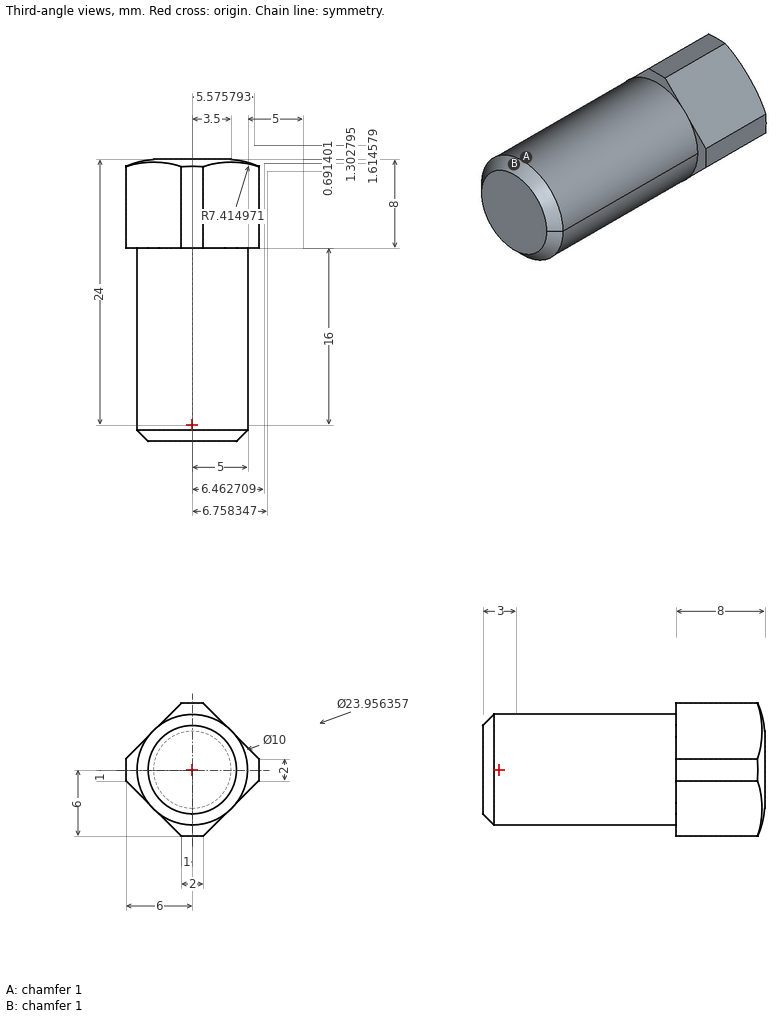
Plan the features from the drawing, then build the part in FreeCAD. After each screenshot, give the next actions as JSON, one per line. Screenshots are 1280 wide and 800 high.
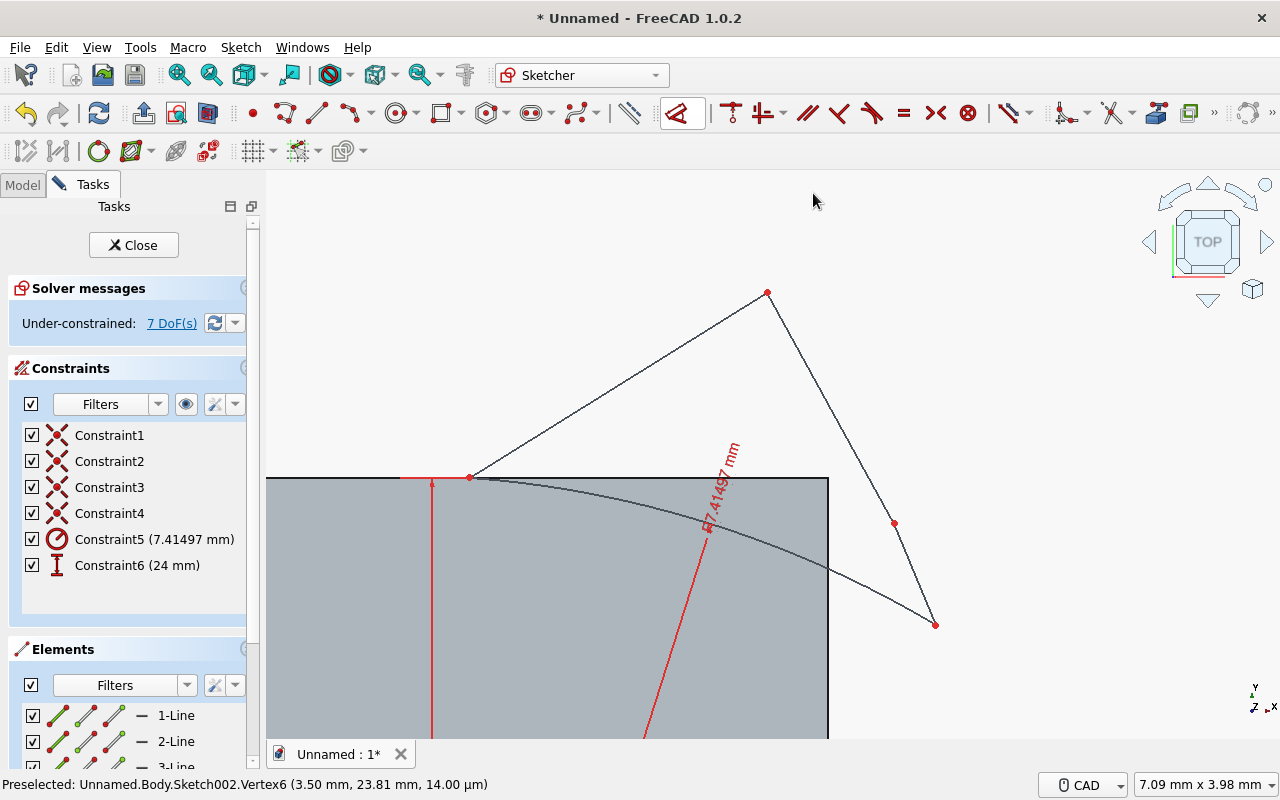
{"action": "left_click", "coordinate": [470, 478]}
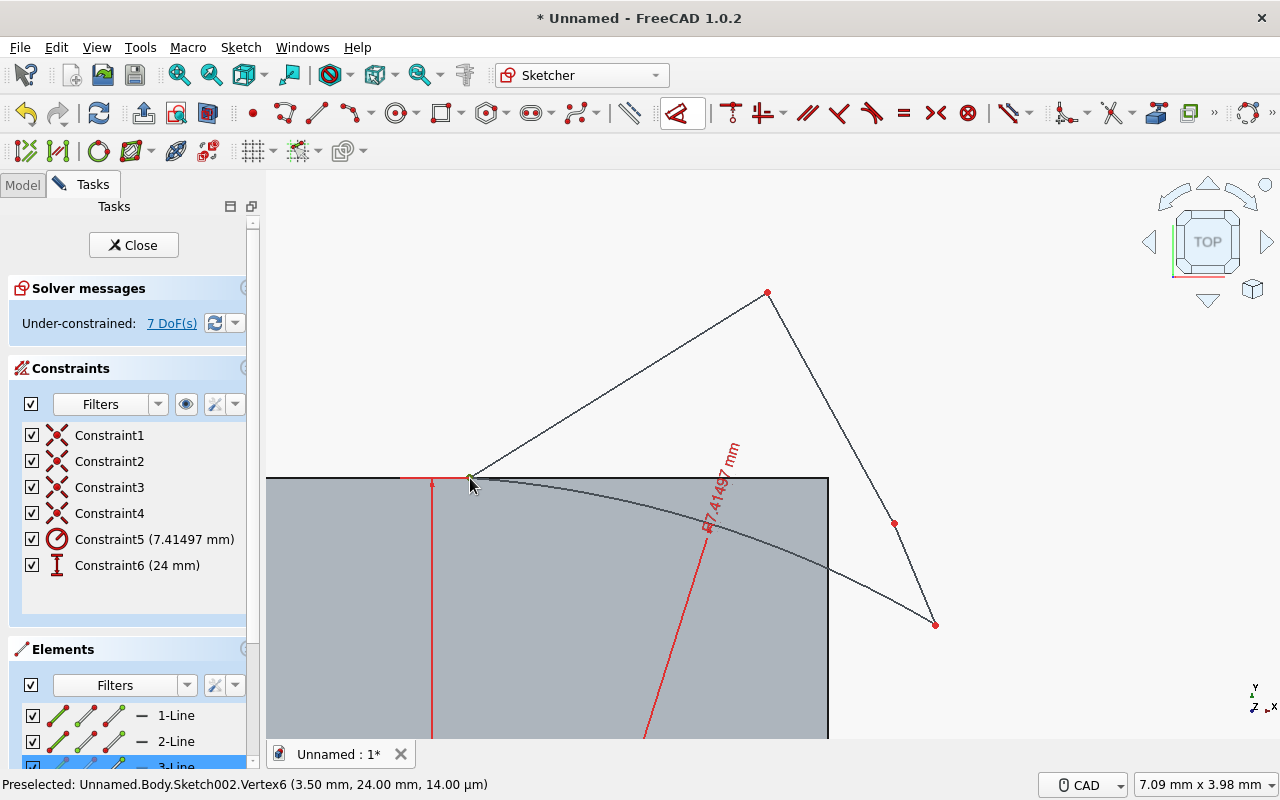
{"action": "left_click", "coordinate": [700, 114]}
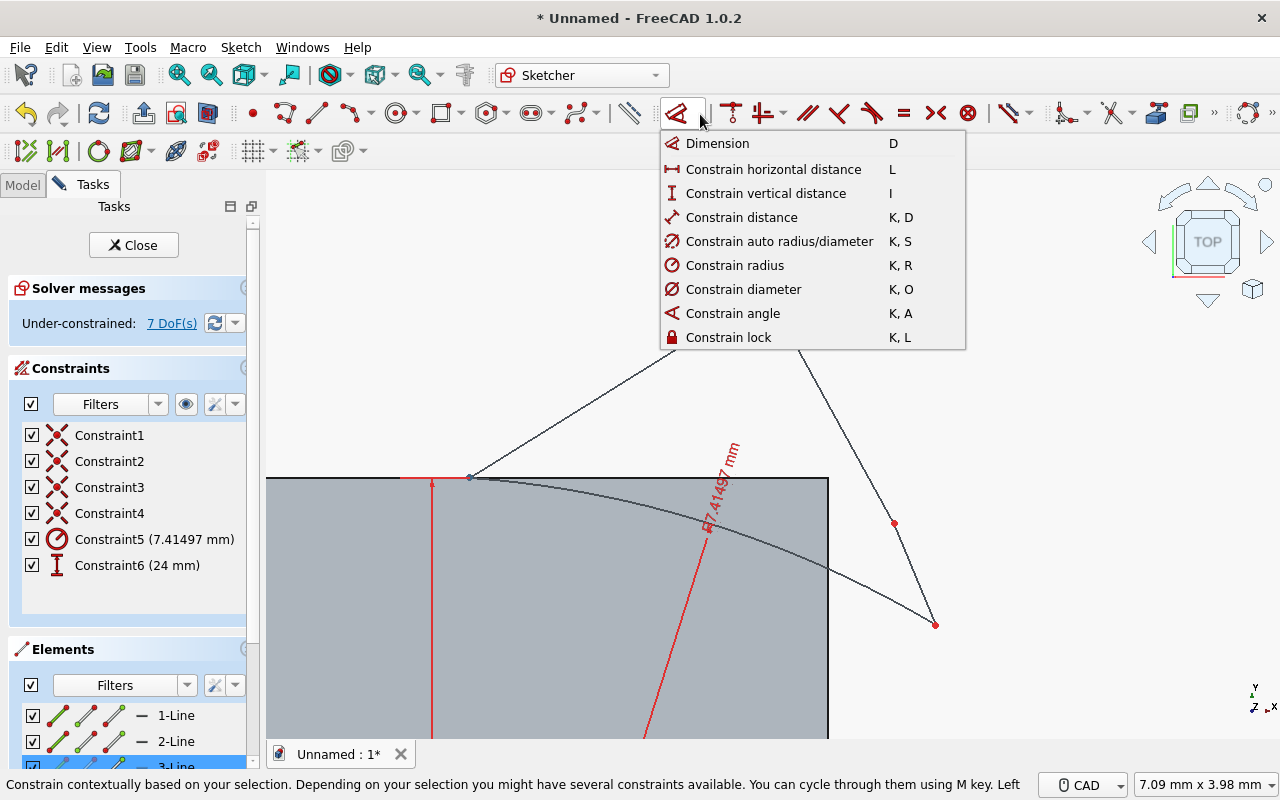
{"action": "left_click", "coordinate": [813, 169]}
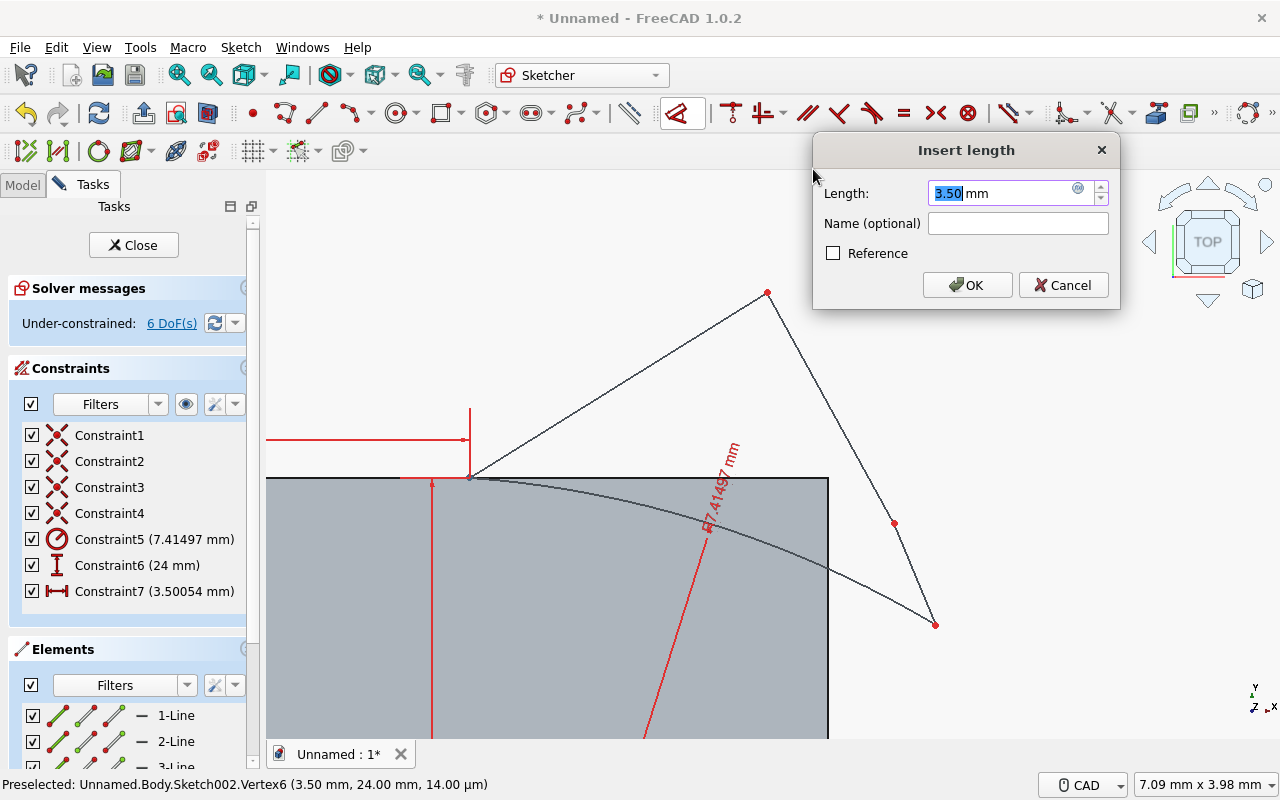
{"action": "type", "text": "3.5"}
{"action": "key", "text": "Return"}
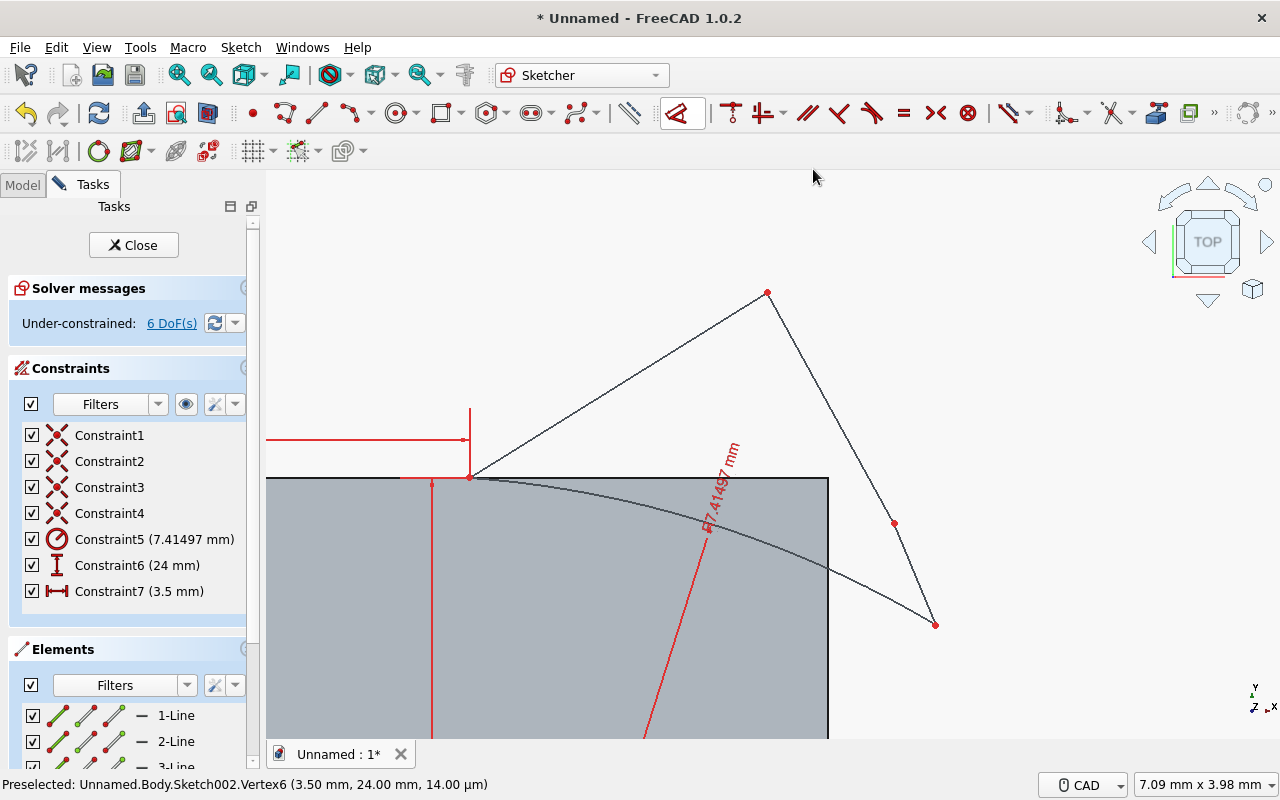
{"action": "left_click", "coordinate": [936, 625]}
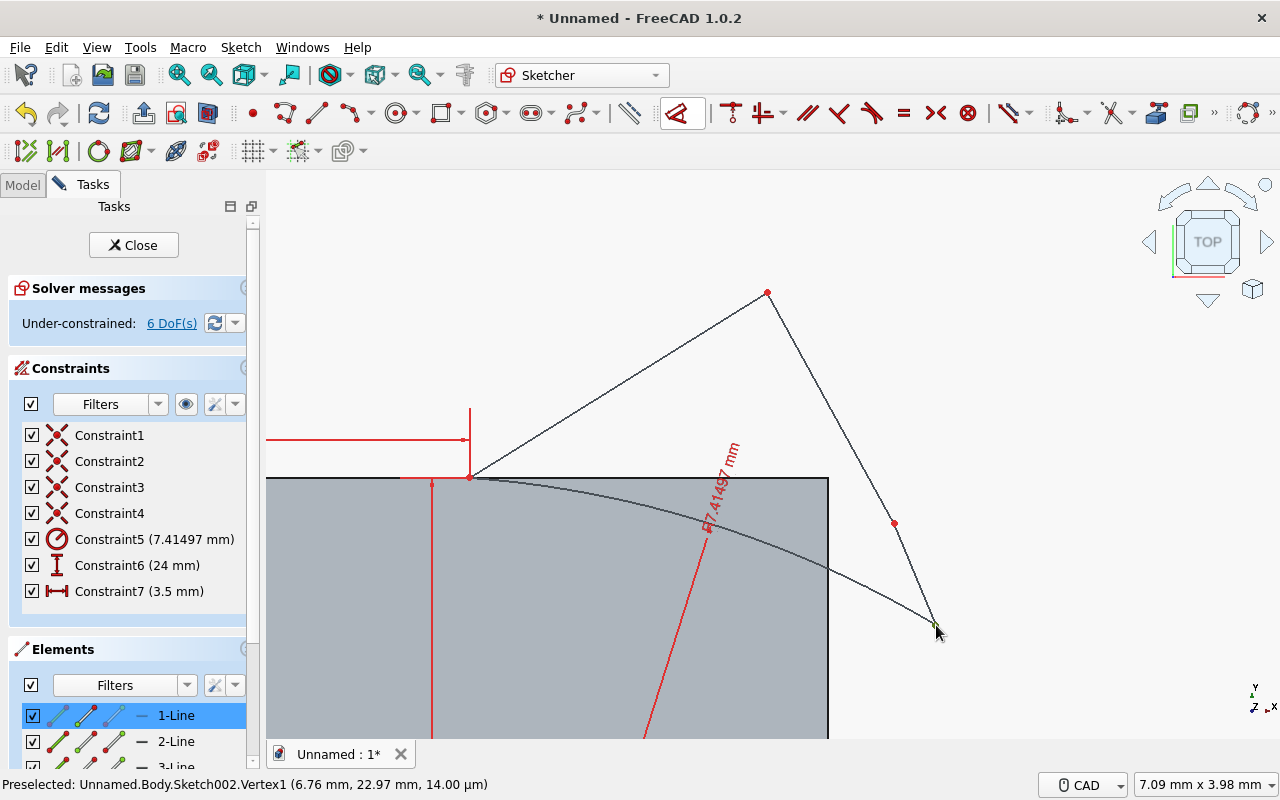
{"action": "left_click", "coordinate": [700, 114]}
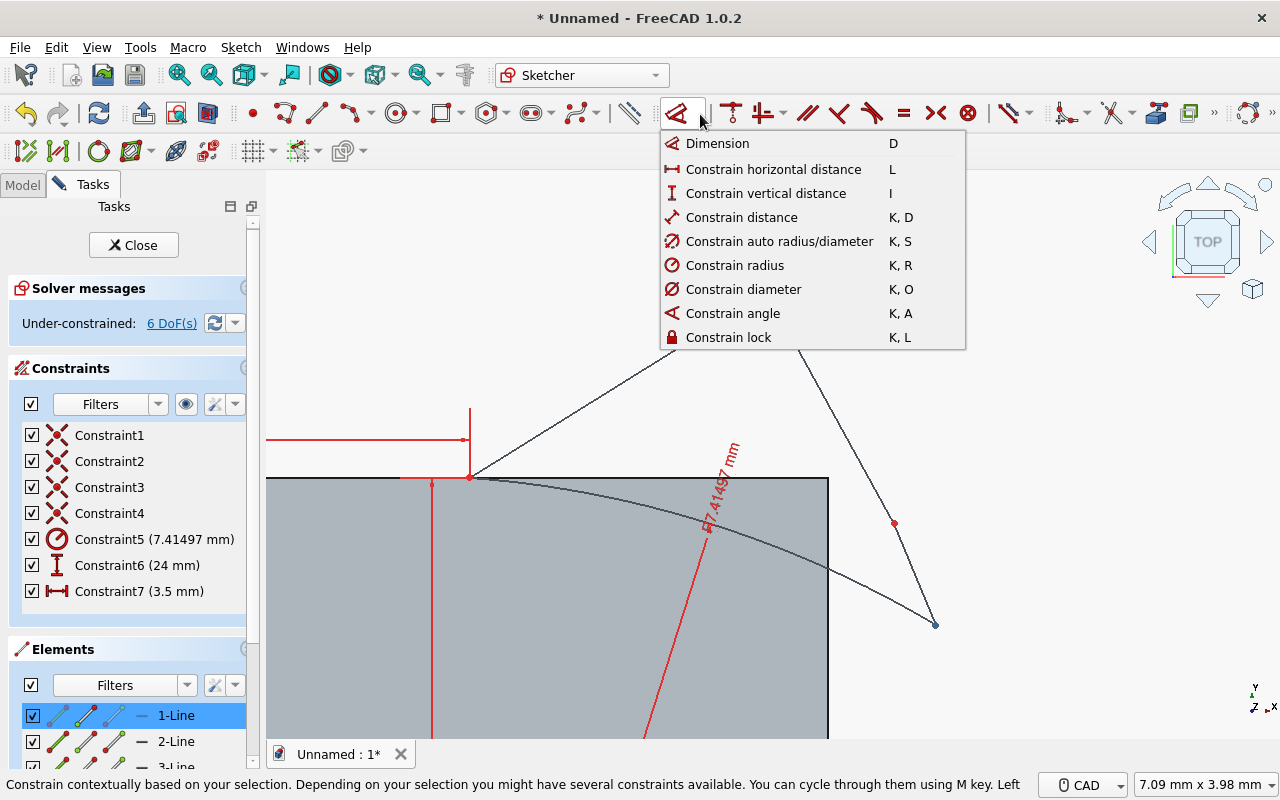
{"action": "left_click", "coordinate": [813, 169]}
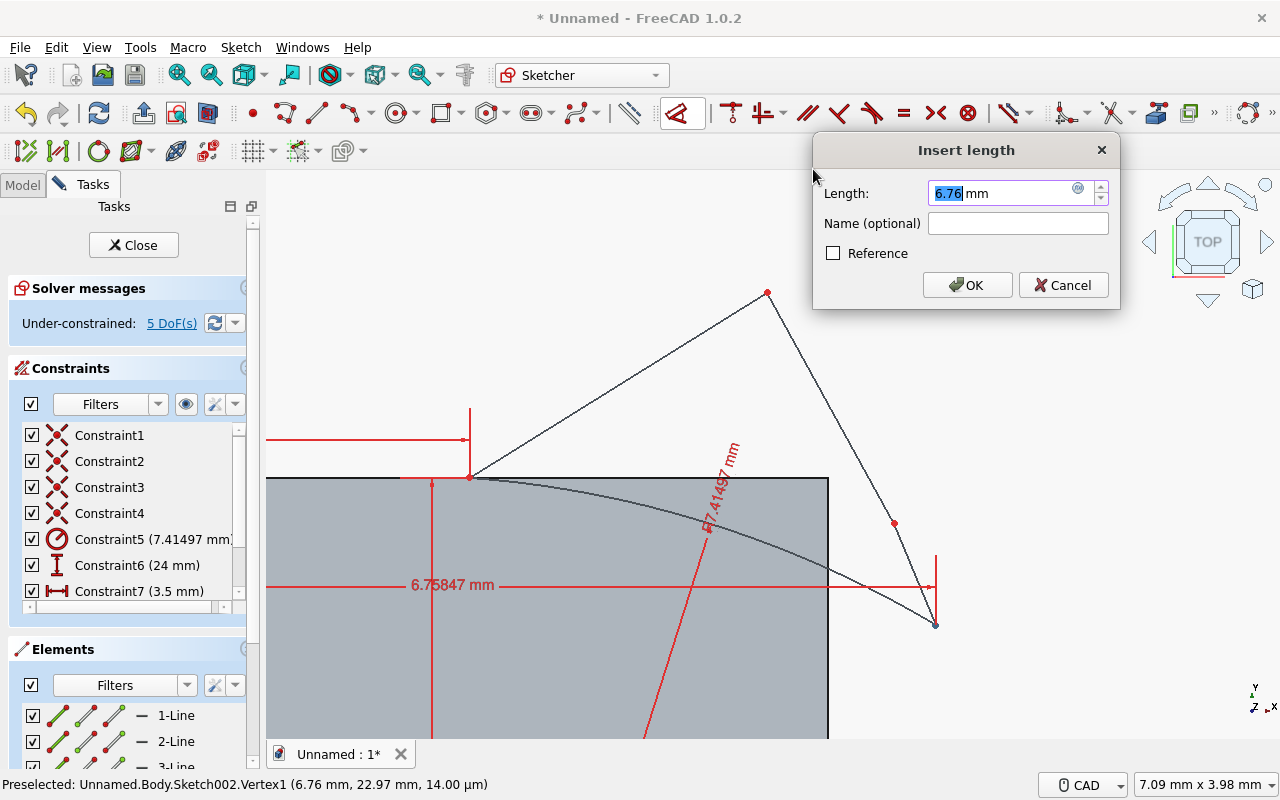
{"action": "type", "text": "6.758347"}
{"action": "key", "text": "Return"}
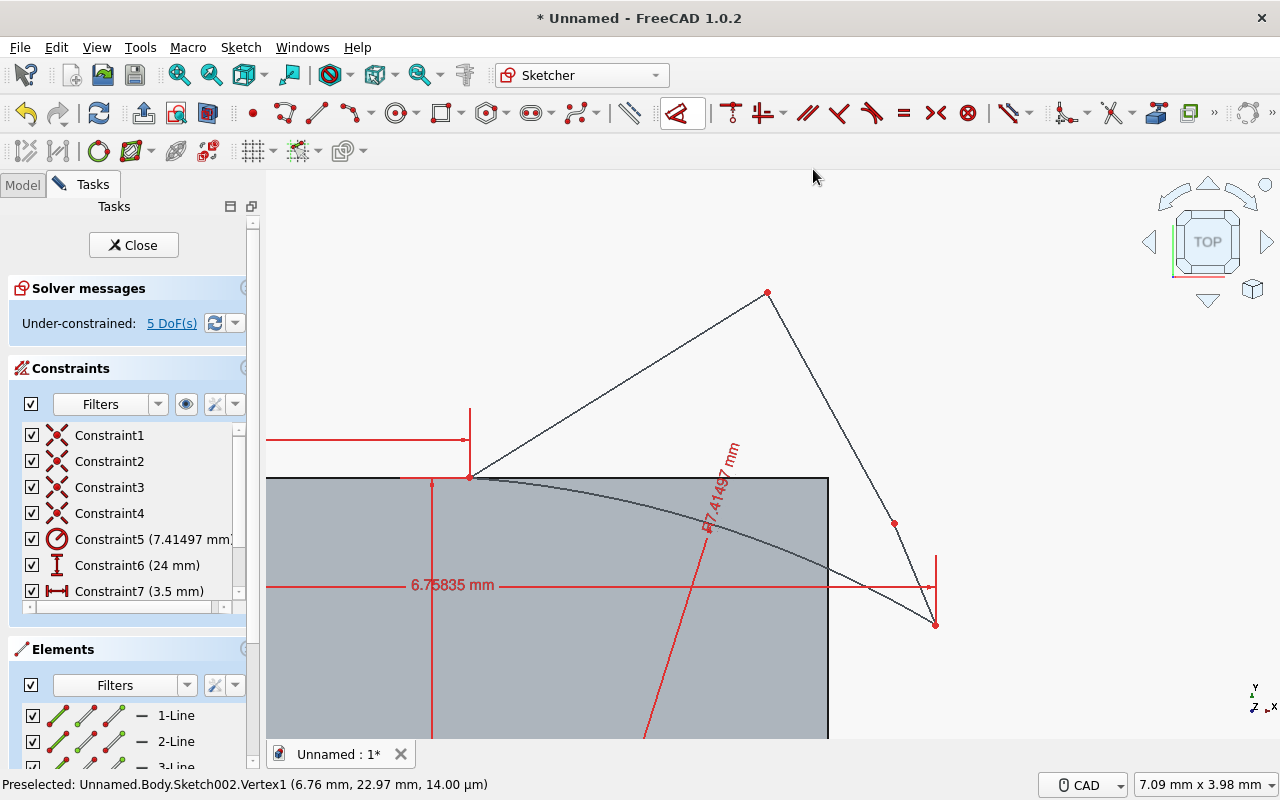
{"action": "left_click", "coordinate": [894, 524]}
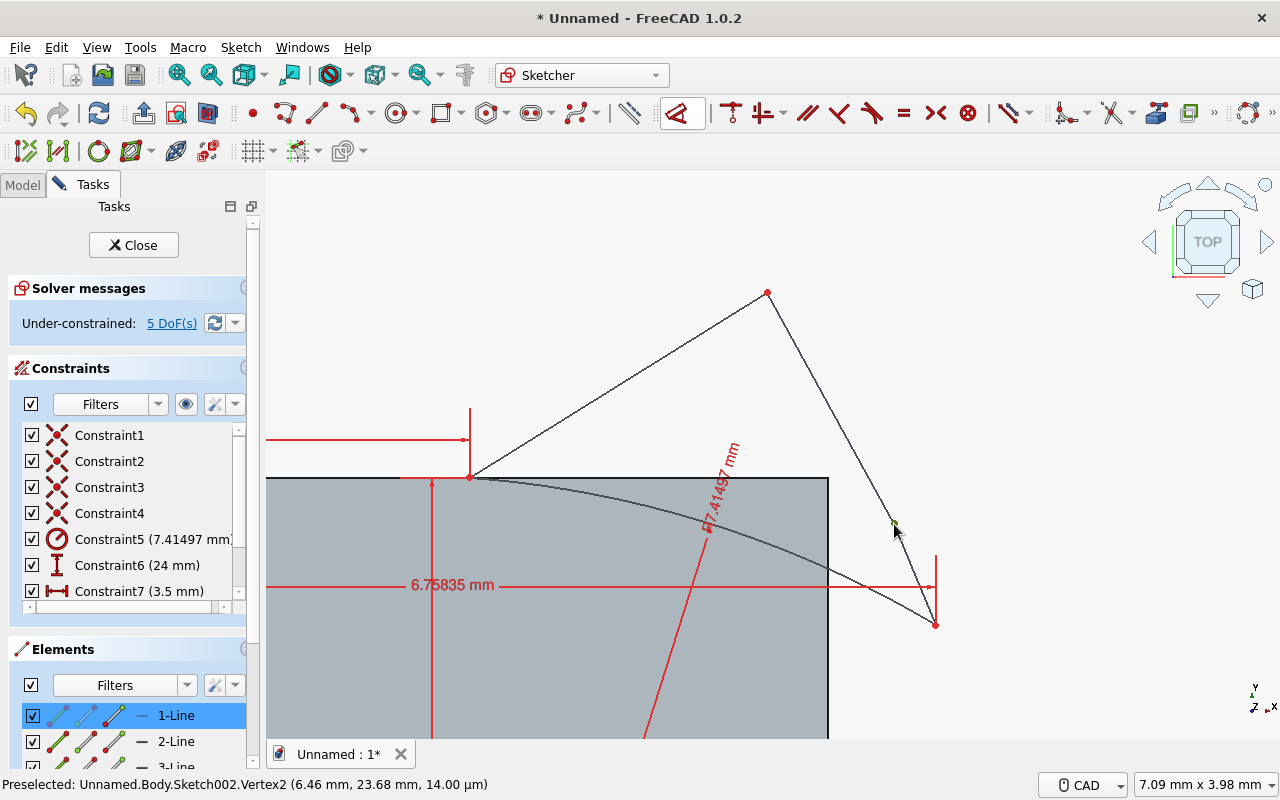
{"action": "left_click", "coordinate": [700, 114]}